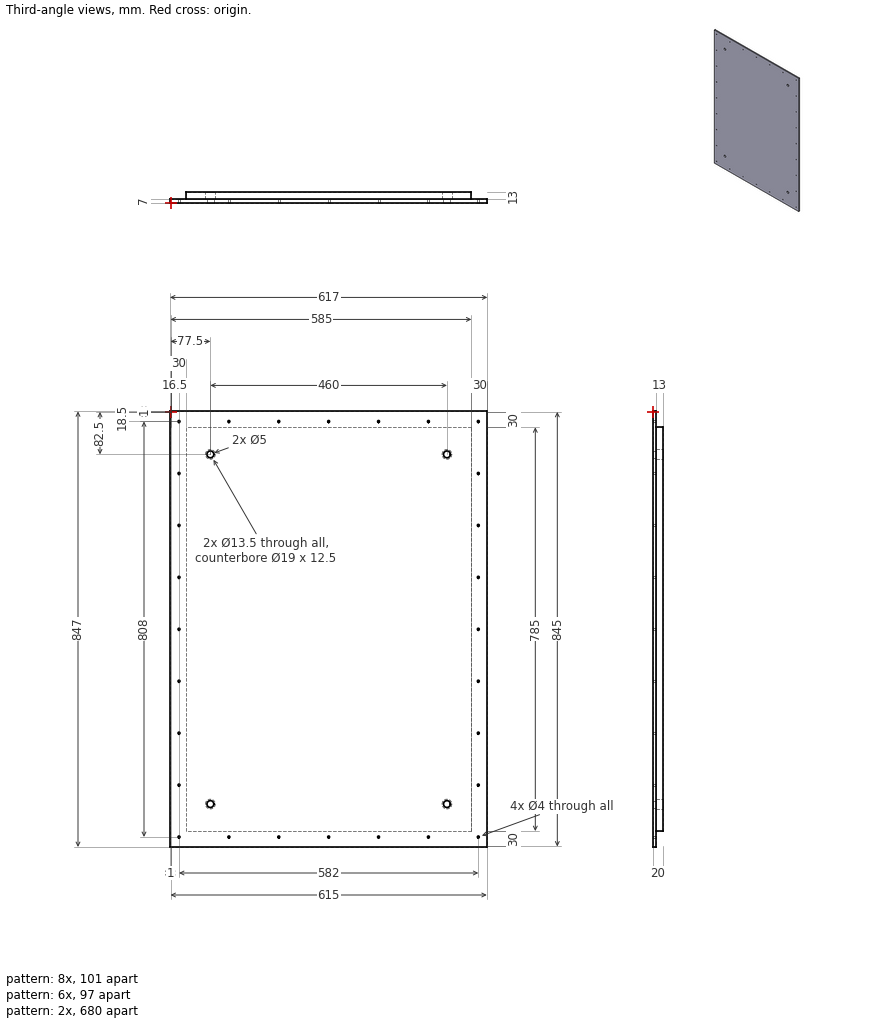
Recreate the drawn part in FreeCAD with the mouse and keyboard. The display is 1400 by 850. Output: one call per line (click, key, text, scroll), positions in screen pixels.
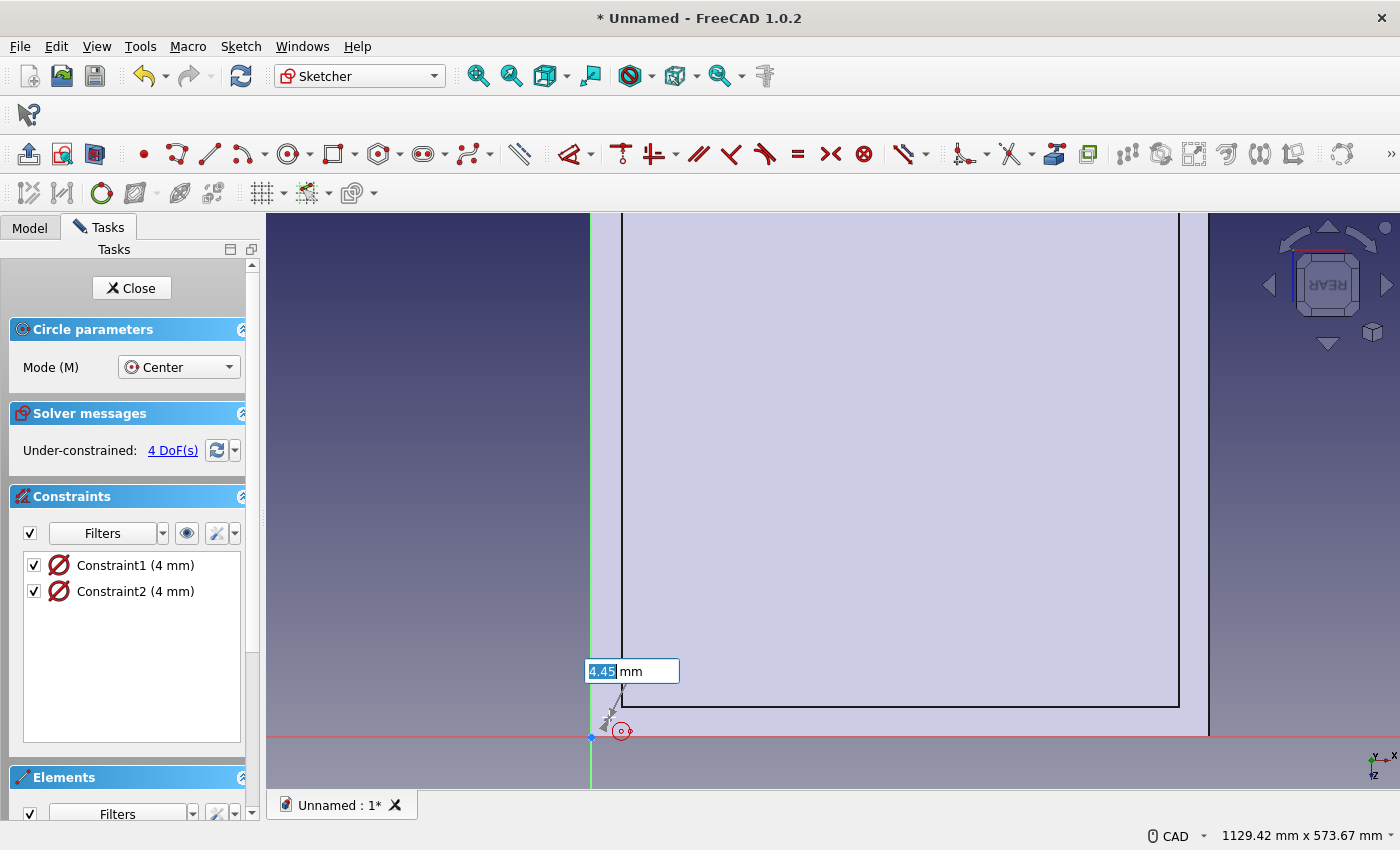
text(4)
key(Return)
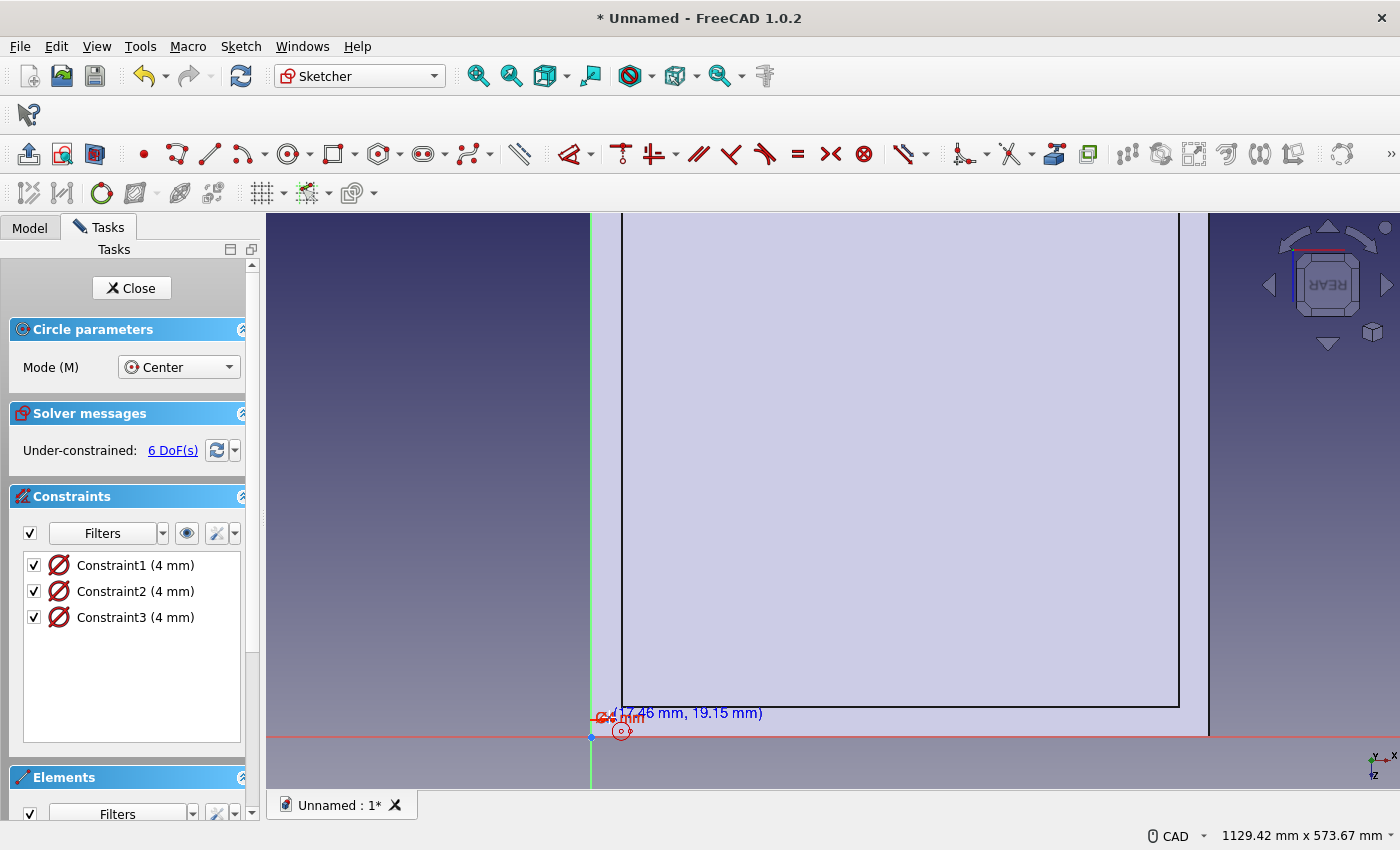
scroll(1192, 719, up, 13)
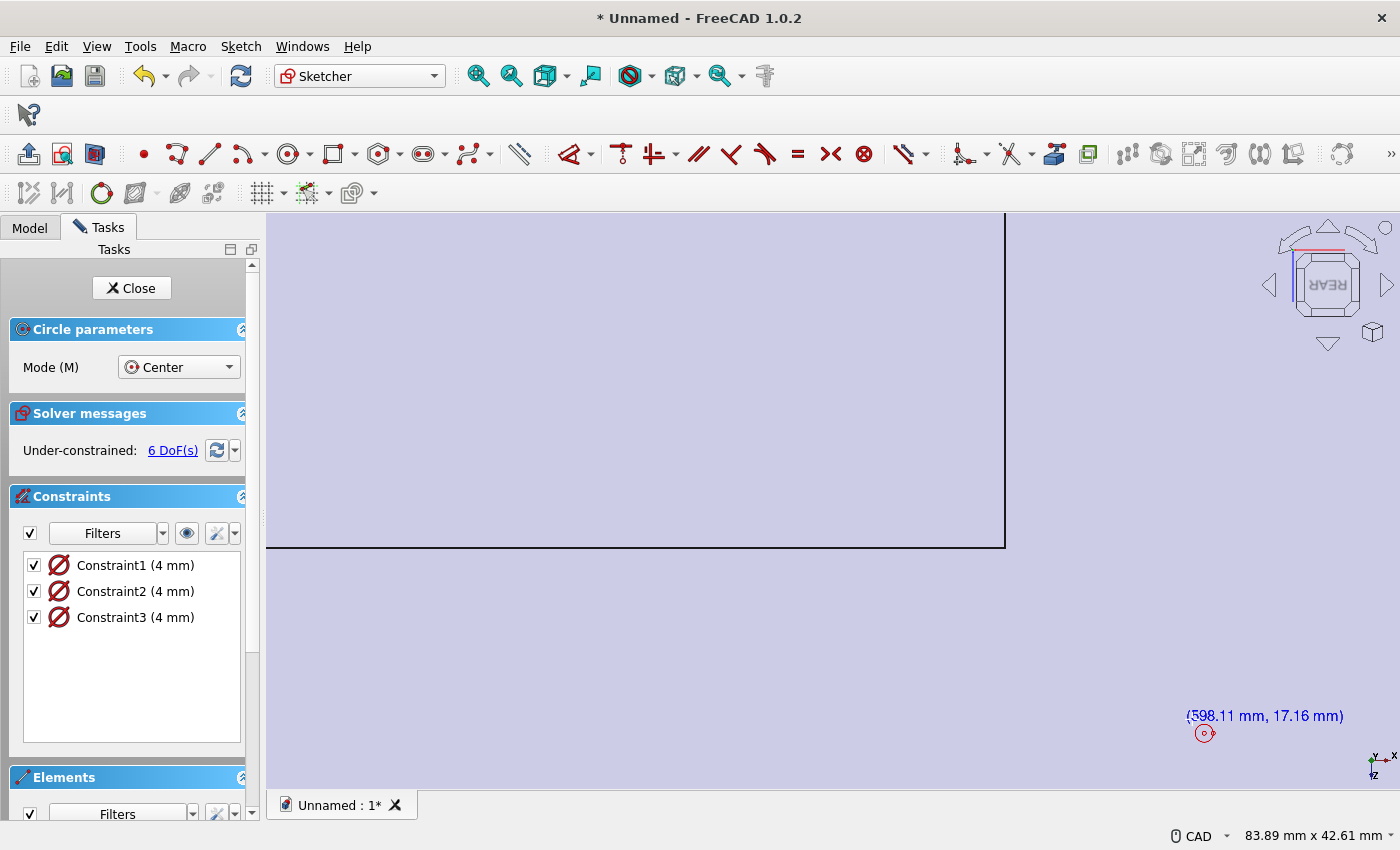
scroll(918, 720, down, 16)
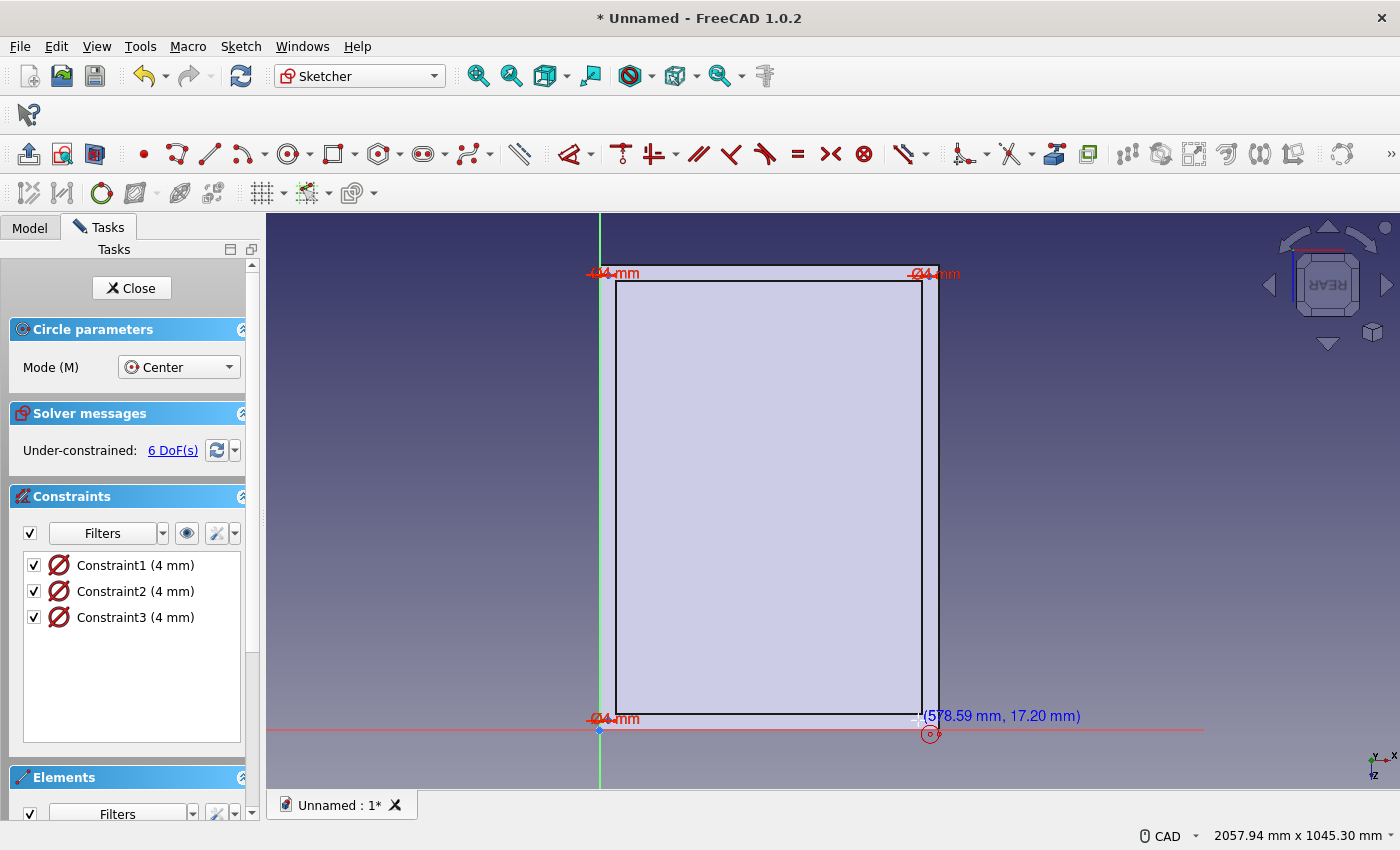
scroll(930, 720, up, 3)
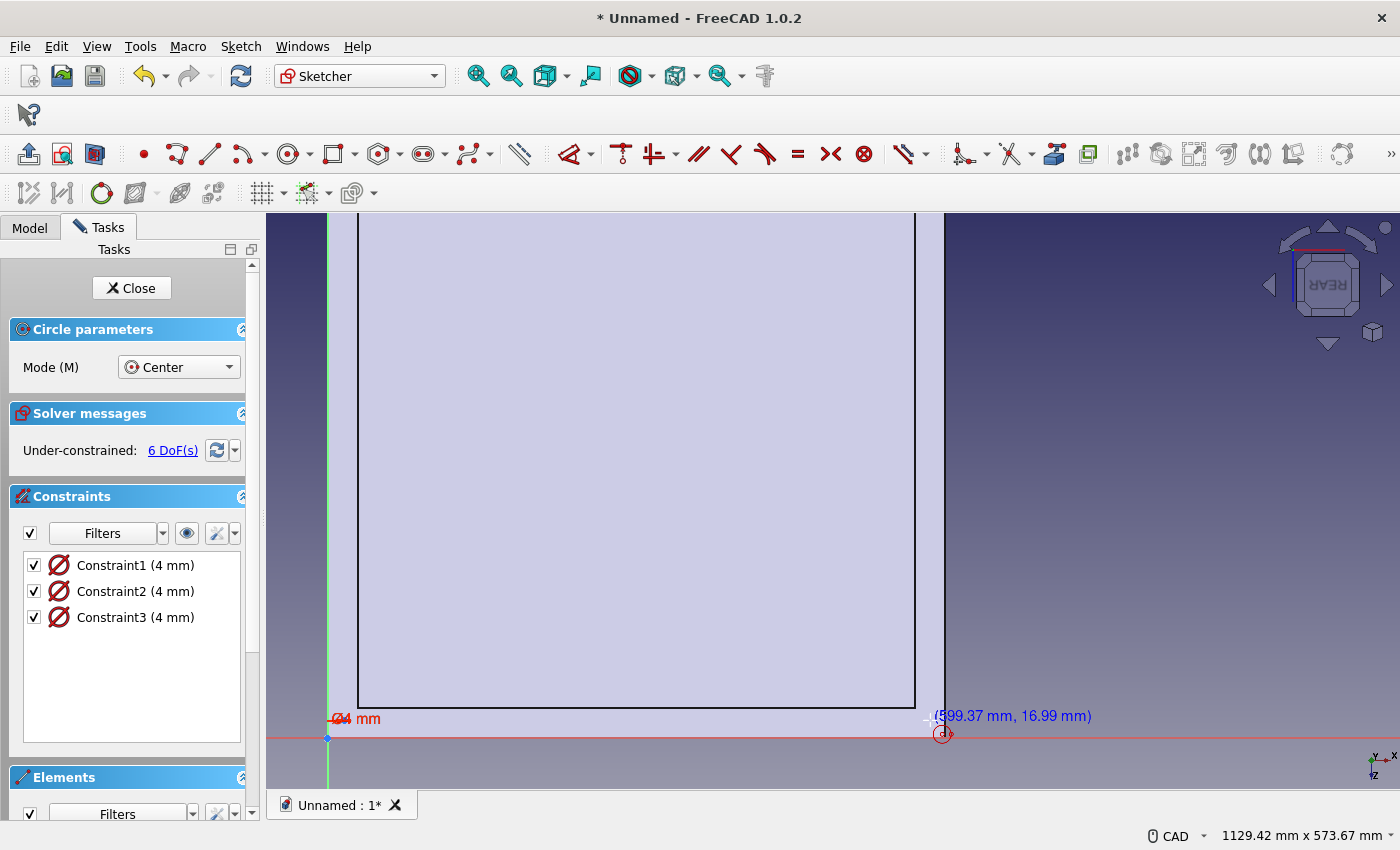
click(929, 720)
move(930, 718)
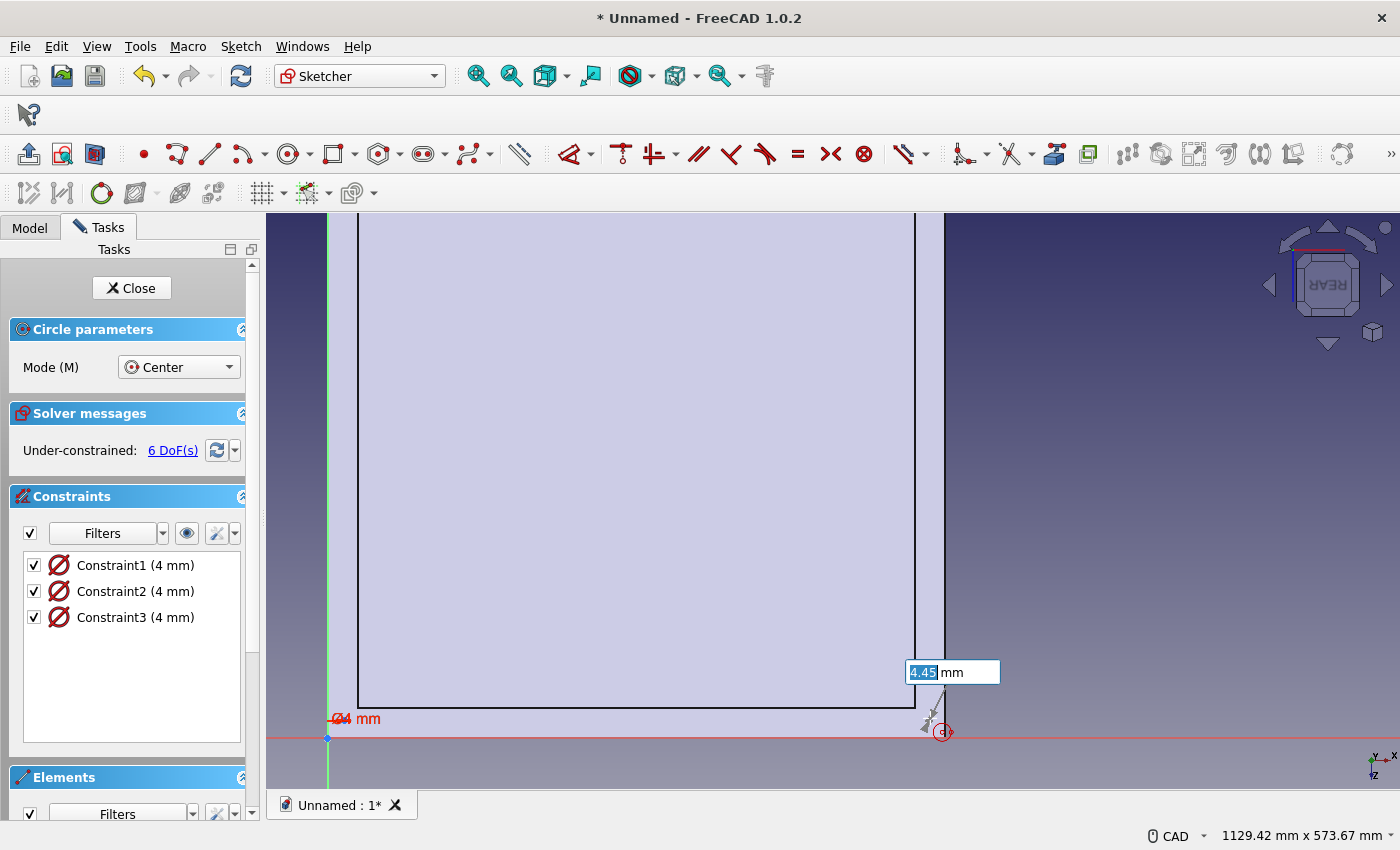
text(4)
key(Return)
key(Escape)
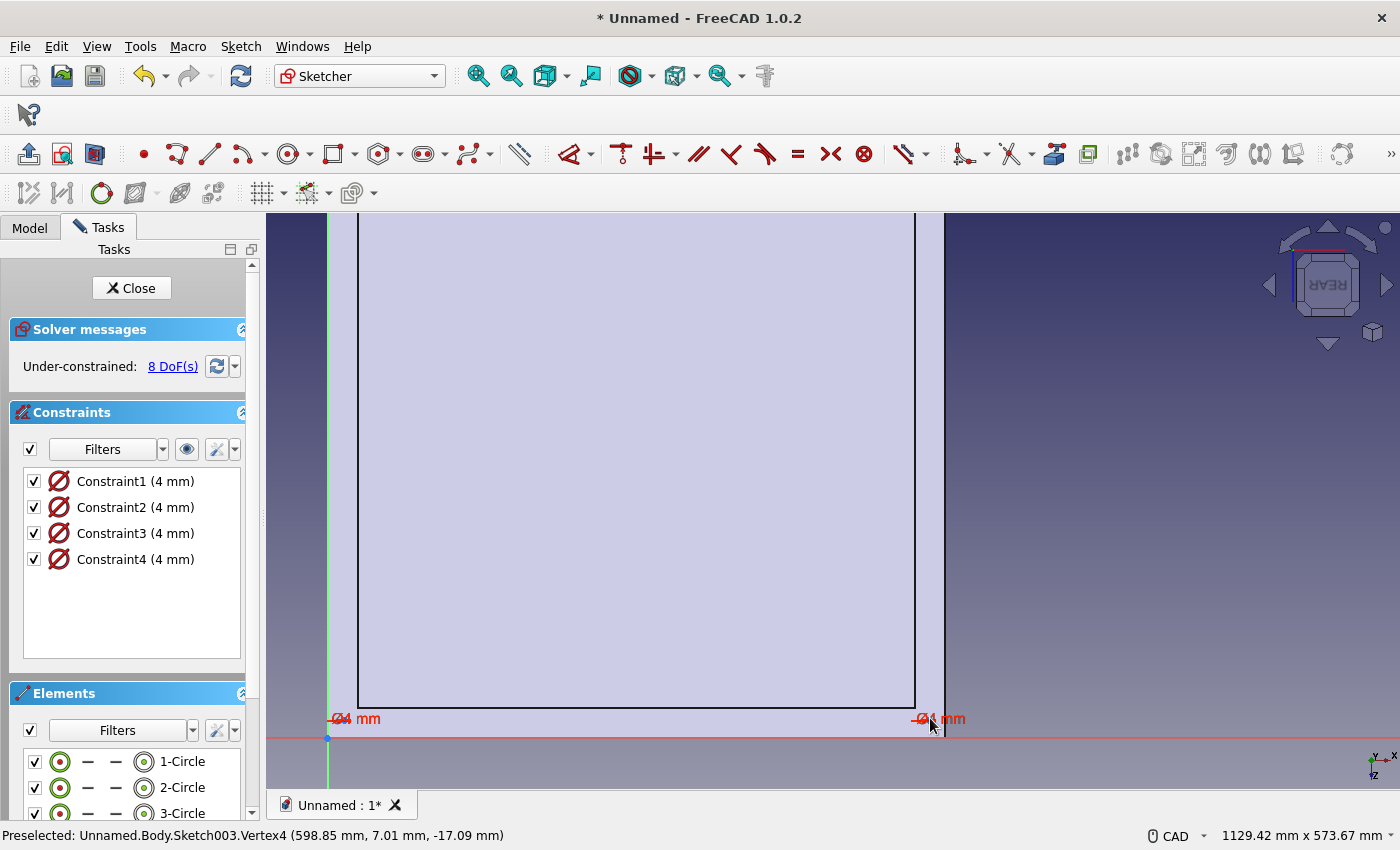
scroll(875, 647, down, 4)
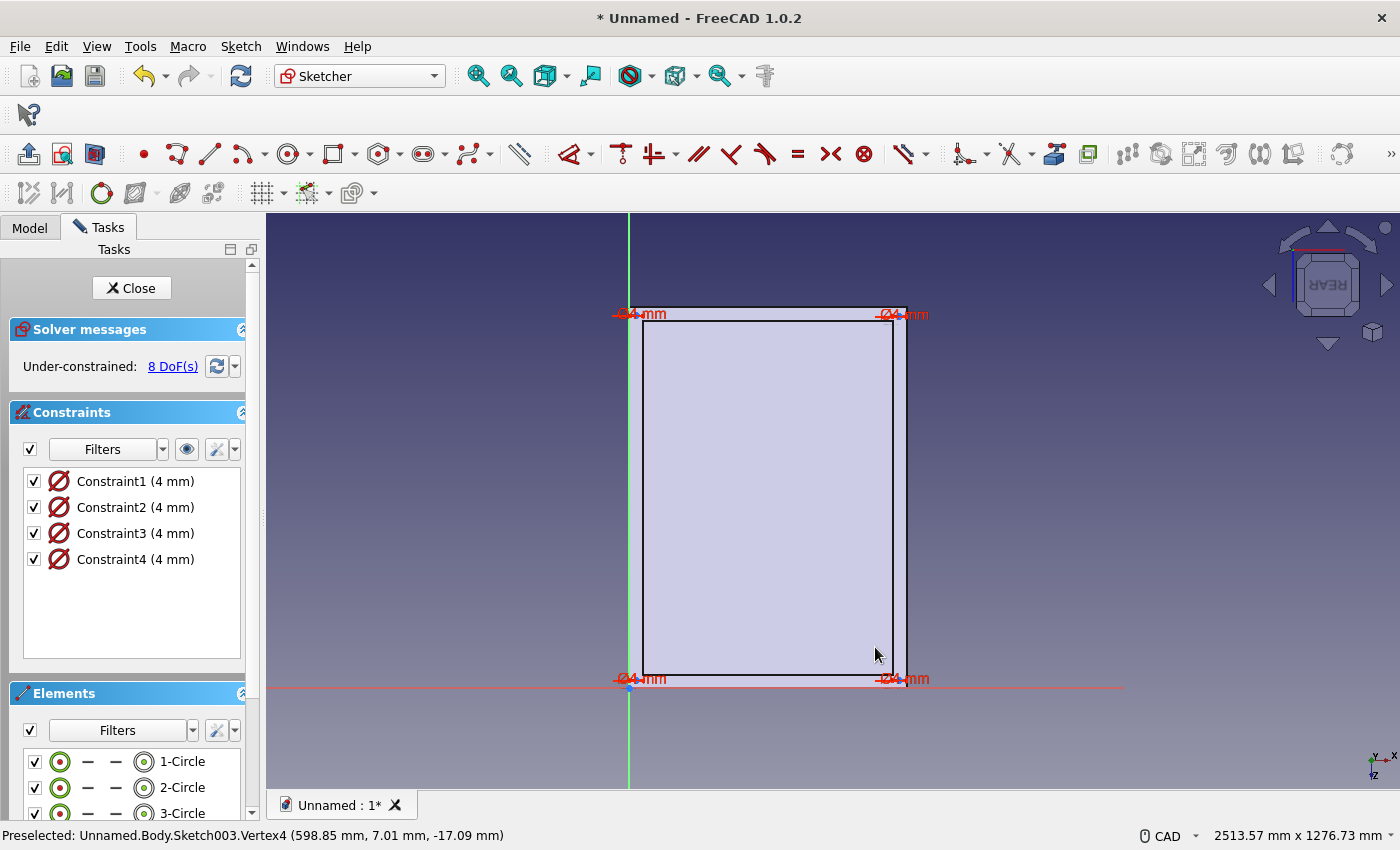
click(899, 317)